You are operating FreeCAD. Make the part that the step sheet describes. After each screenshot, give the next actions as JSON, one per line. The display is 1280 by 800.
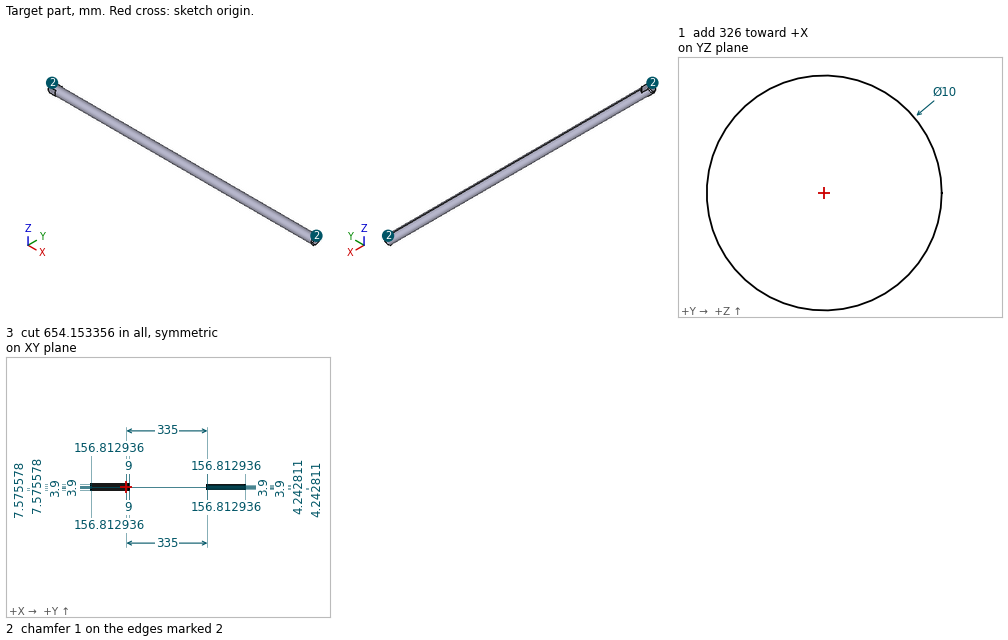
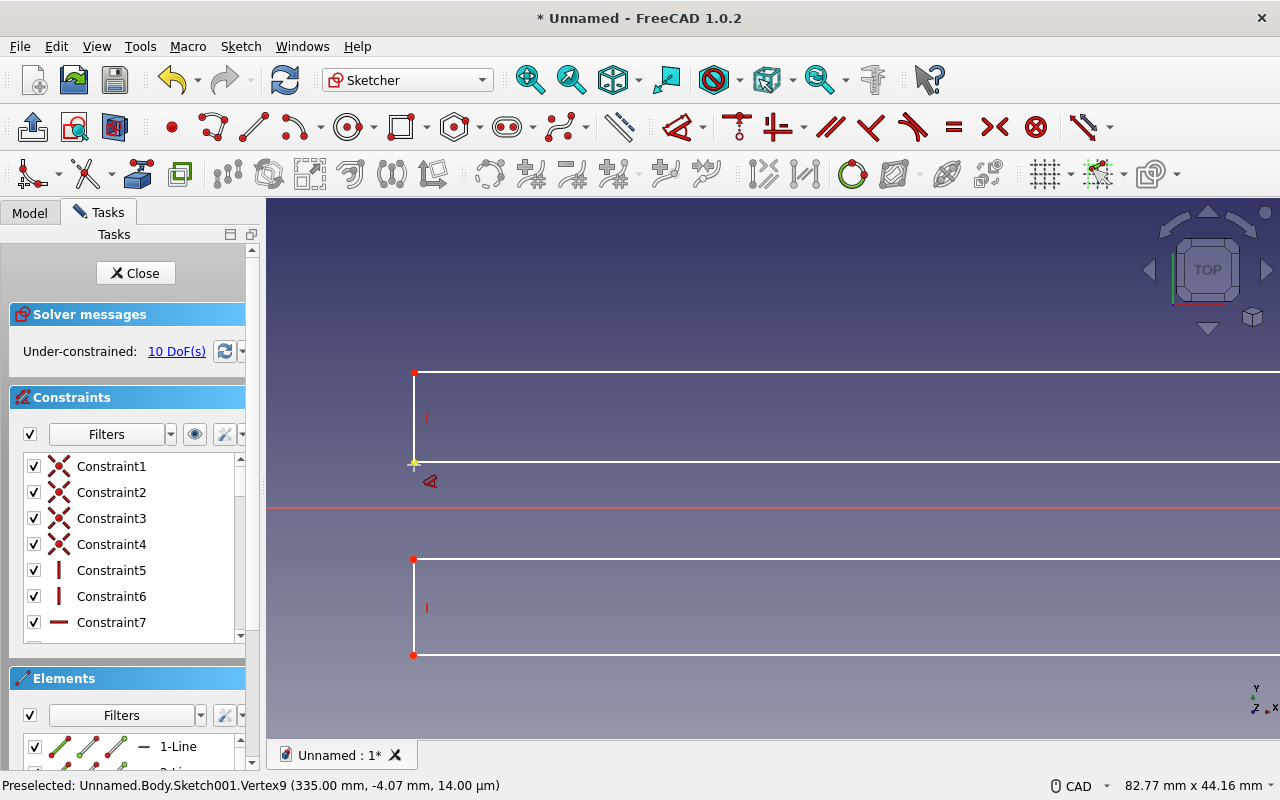
{"action": "left_click", "coordinate": [414, 462]}
{"action": "left_click", "coordinate": [380, 485]}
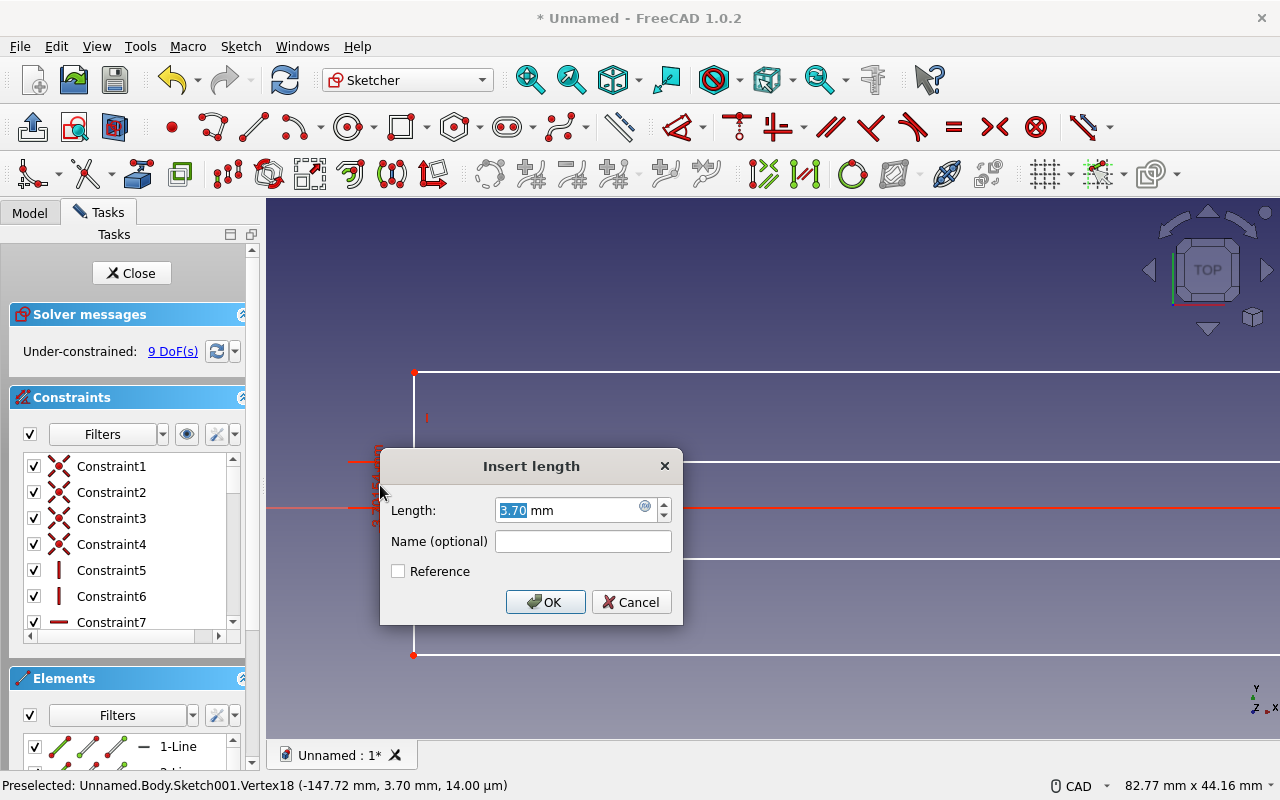
{"action": "type", "text": "3.9"}
{"action": "key", "text": "Return"}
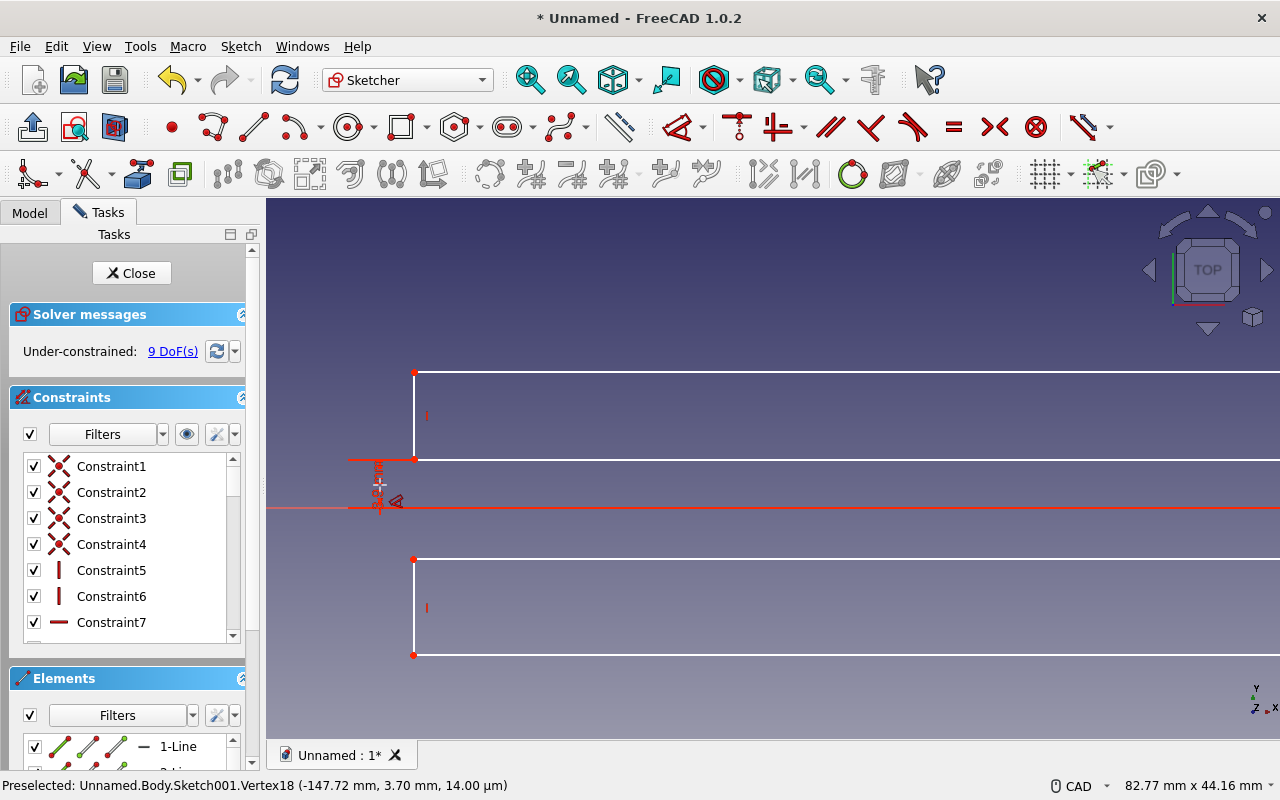
{"action": "left_click", "coordinate": [414, 559]}
{"action": "left_click", "coordinate": [380, 533]}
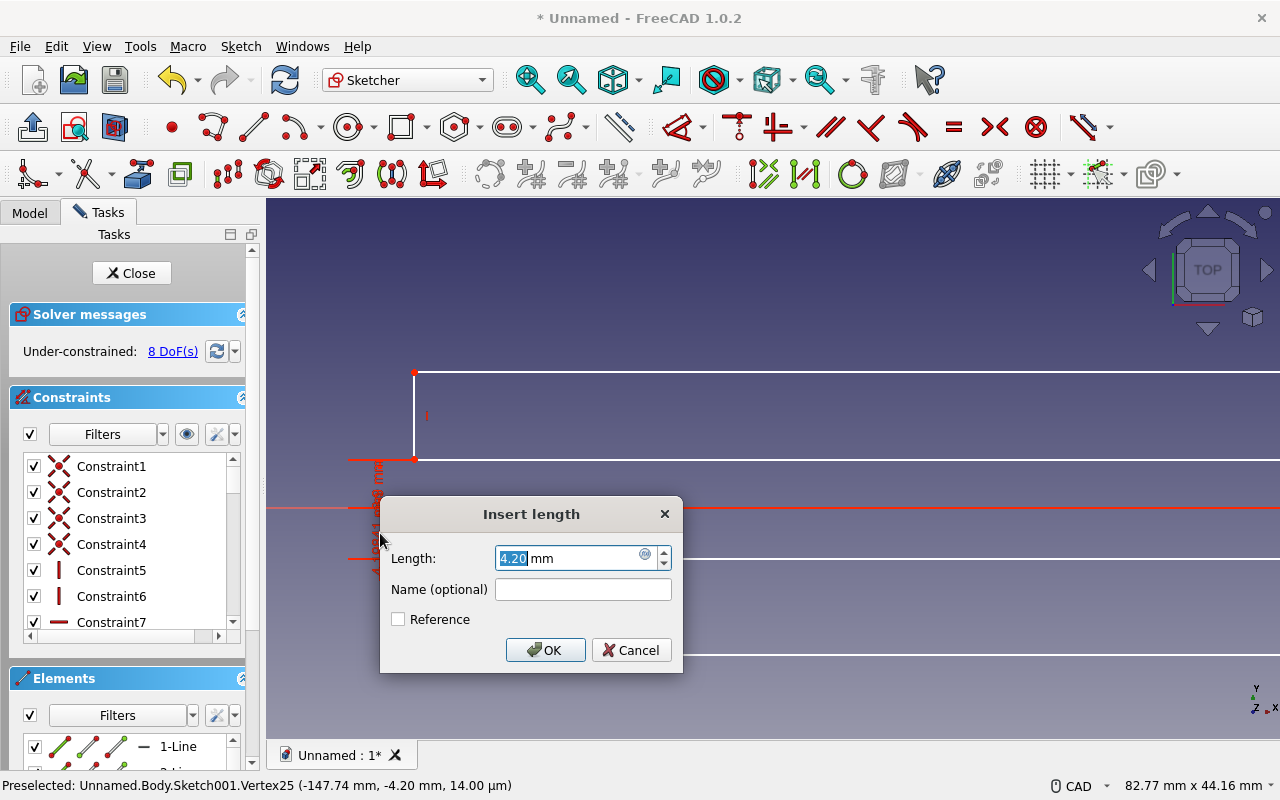
{"action": "type", "text": "3.9"}
{"action": "key", "text": "Return"}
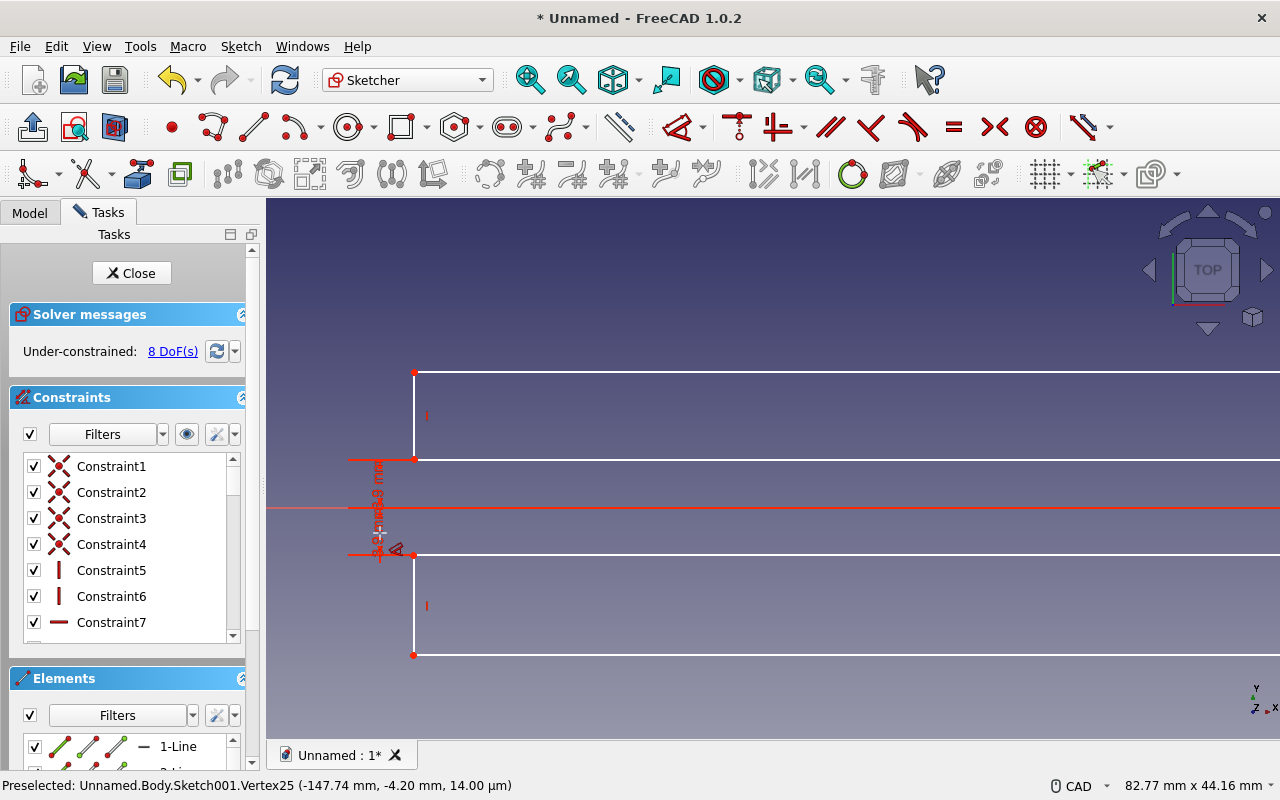
{"action": "scroll", "coordinate": [414, 465], "scroll_direction": "down", "scroll_amount": 13}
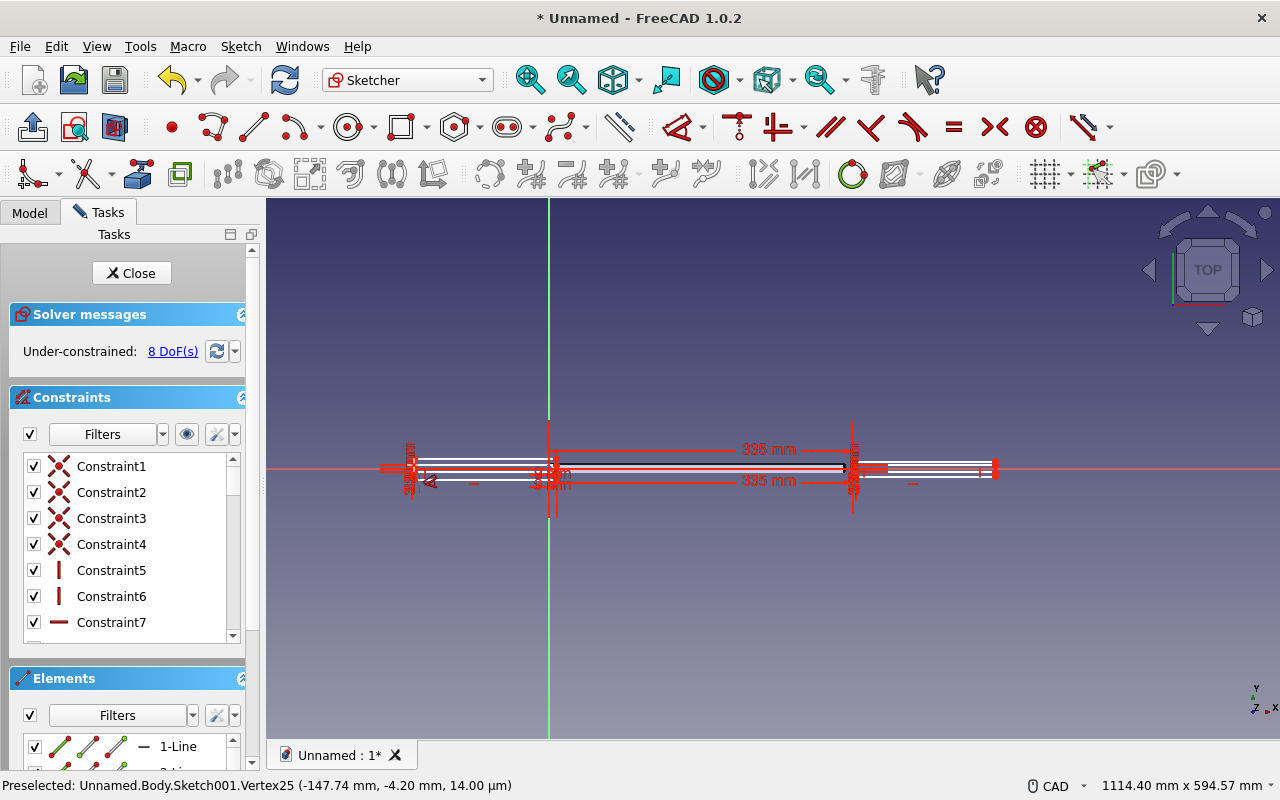
{"action": "scroll", "coordinate": [853, 463], "scroll_direction": "up", "scroll_amount": 13}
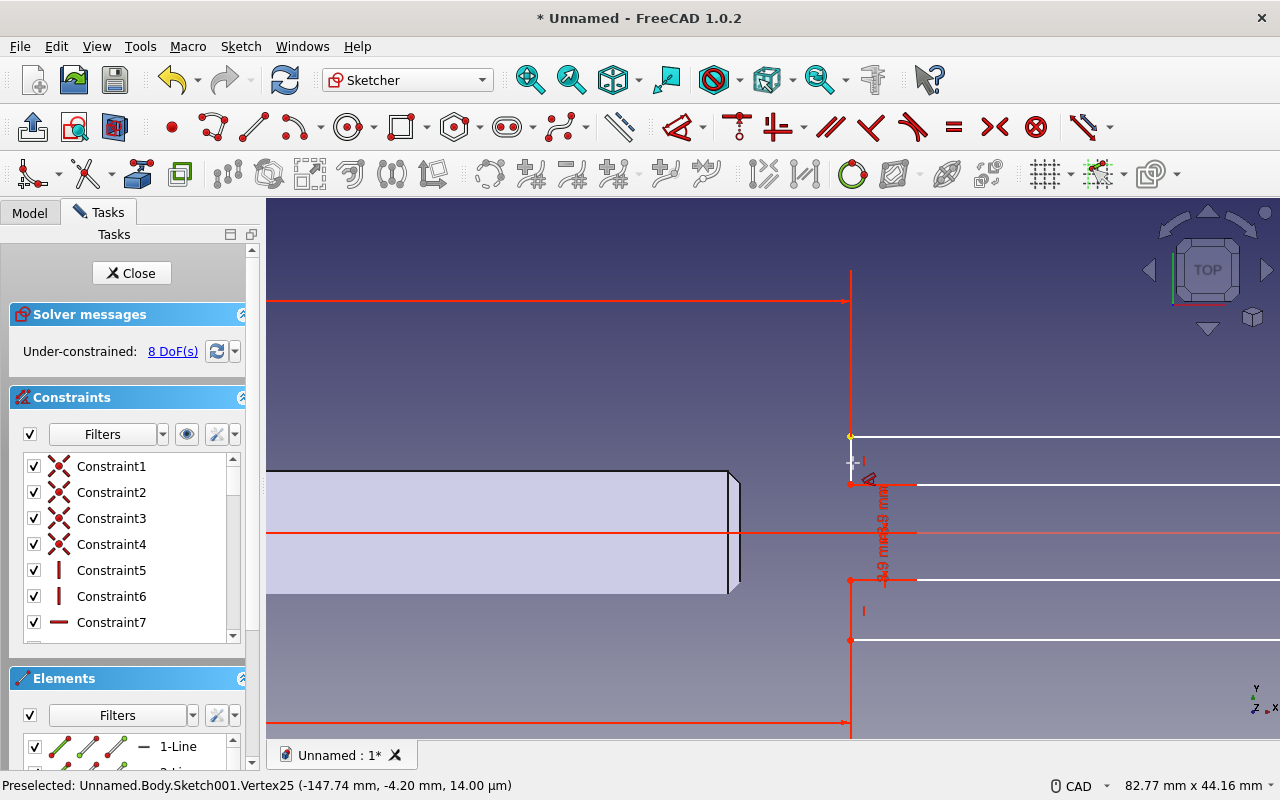
{"action": "left_click", "coordinate": [851, 451]}
{"action": "left_click", "coordinate": [885, 461]}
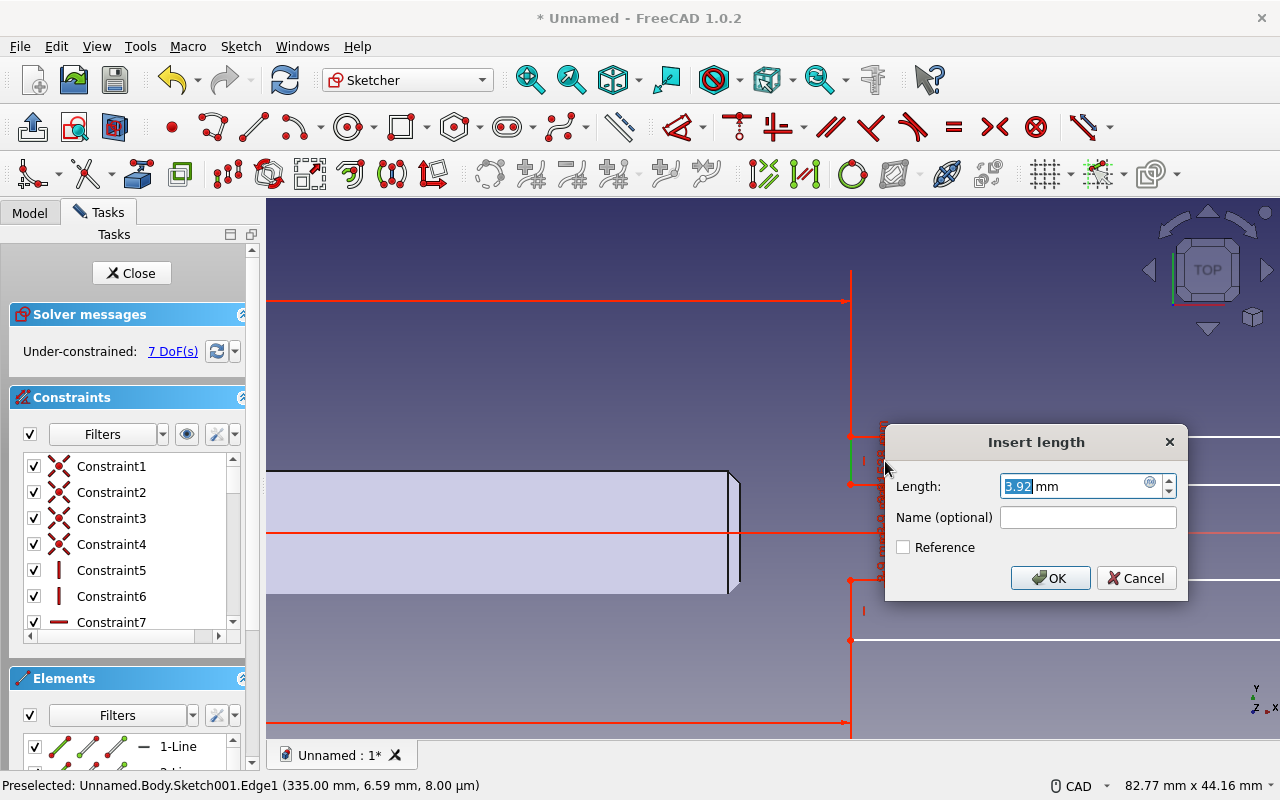
{"action": "type", "text": "4.242811"}
{"action": "key", "text": "Return"}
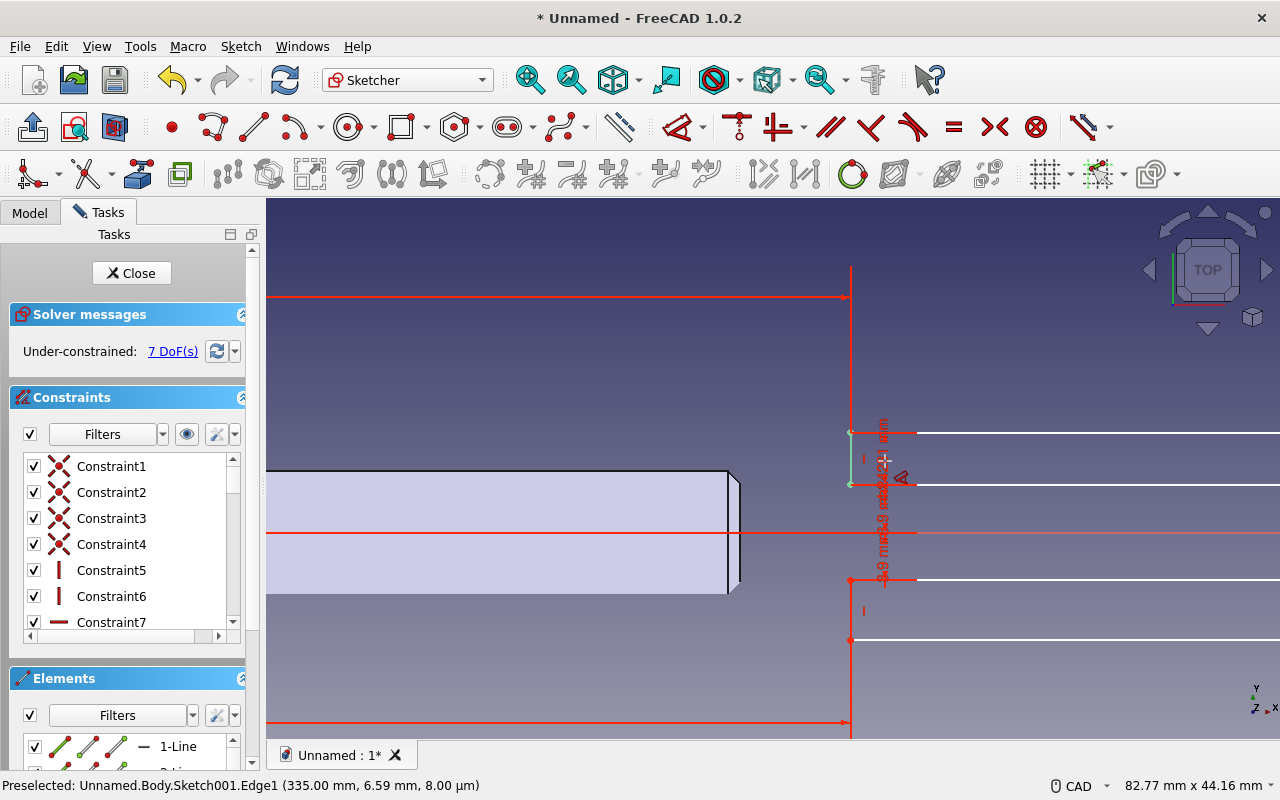
{"action": "left_click", "coordinate": [851, 598]}
{"action": "left_click", "coordinate": [885, 610]}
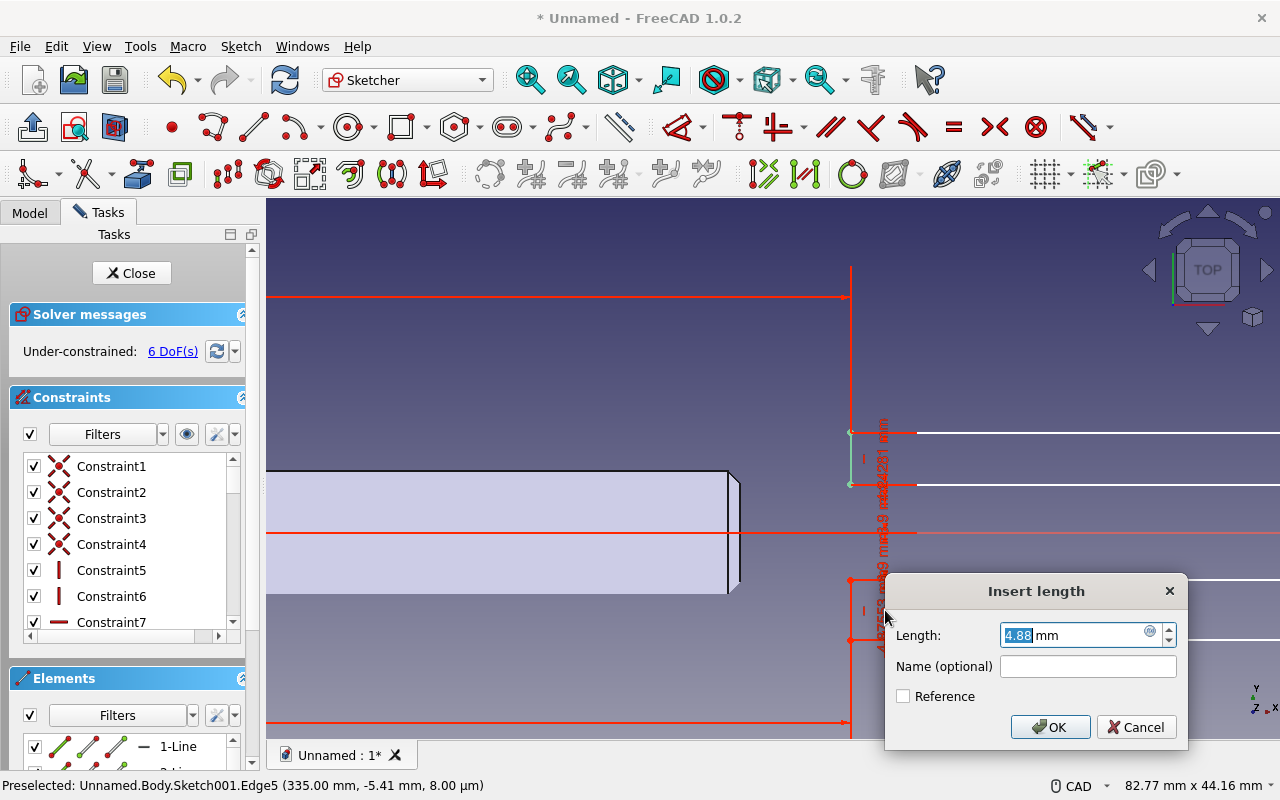
{"action": "type", "text": "4.242811"}
{"action": "key", "text": "Return"}